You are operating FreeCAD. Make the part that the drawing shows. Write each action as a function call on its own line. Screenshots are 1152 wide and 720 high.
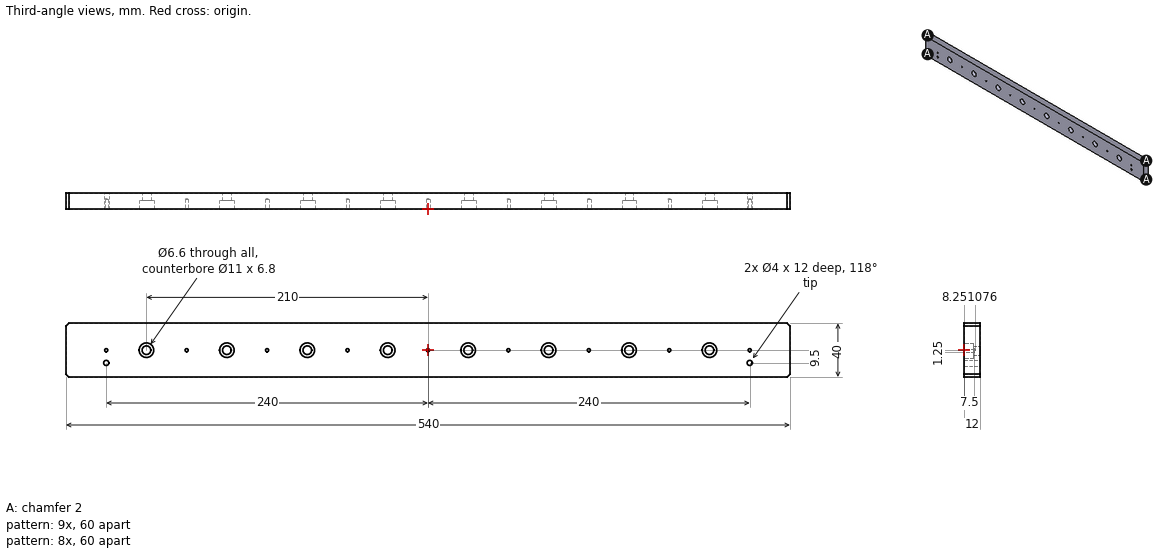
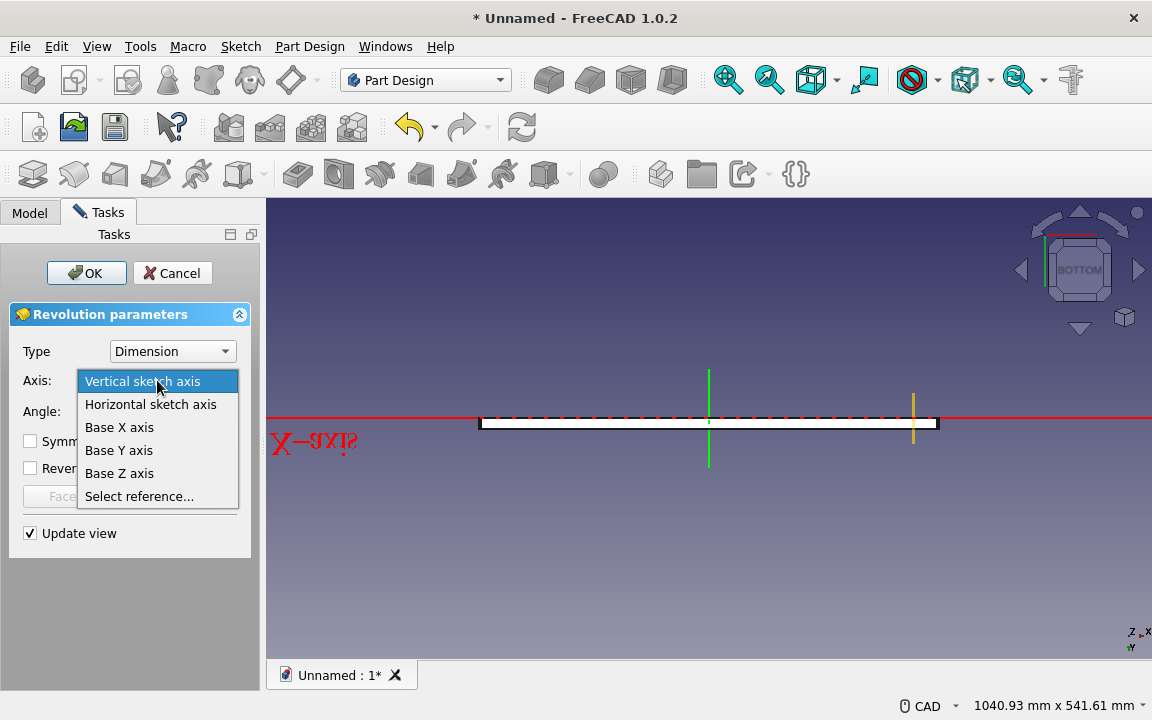
click(156, 404)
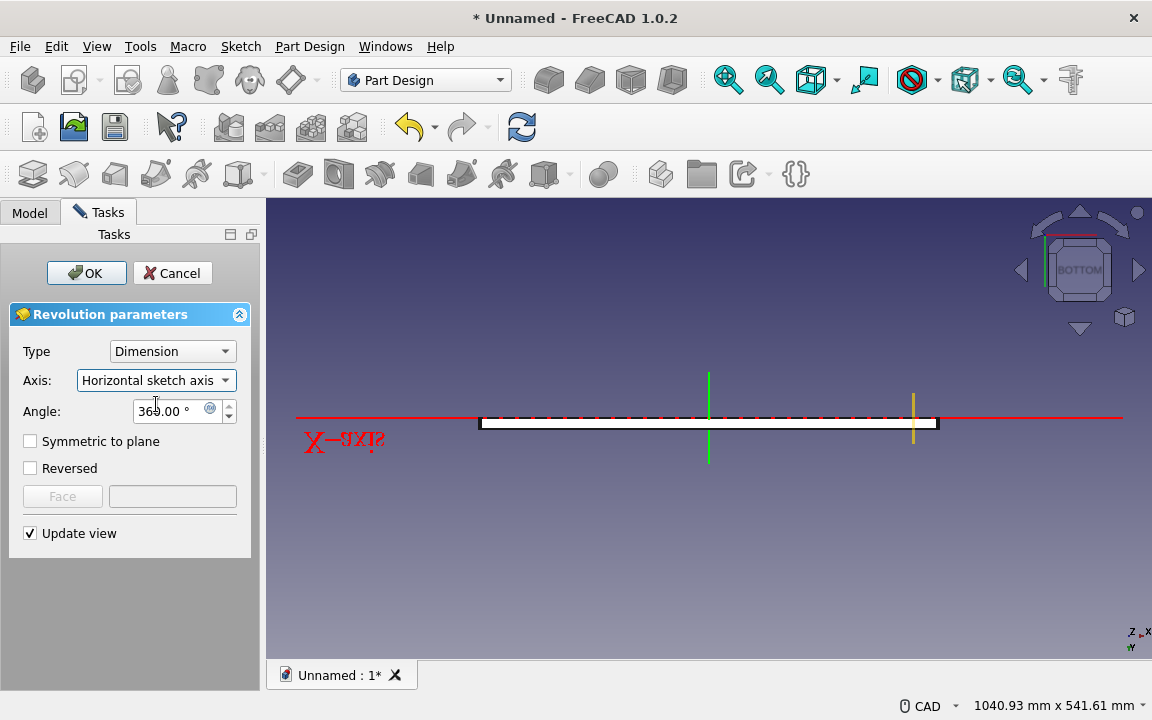
click(87, 273)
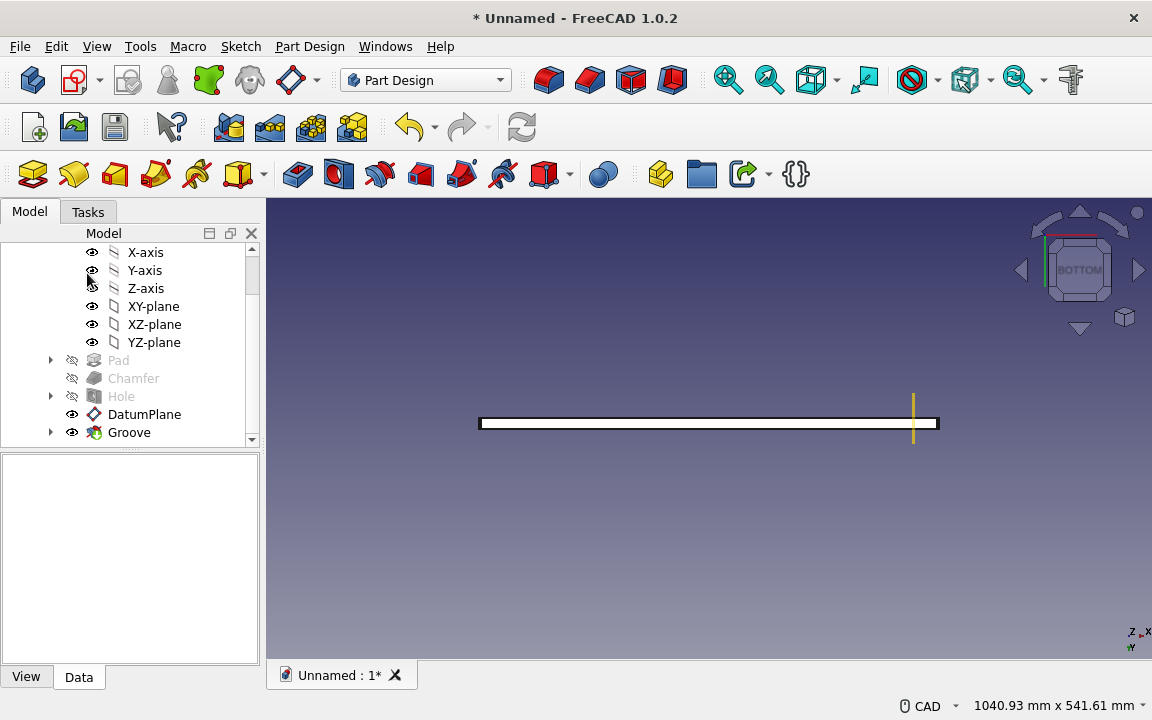
click(117, 414)
key(space)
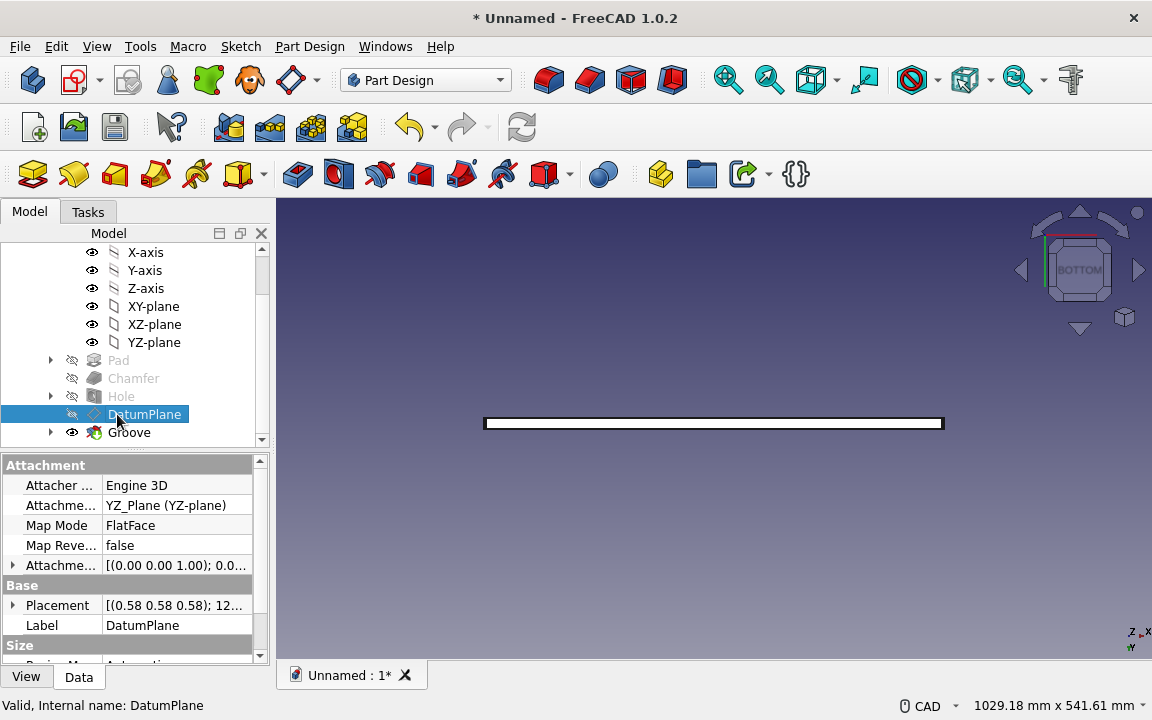
click(117, 432)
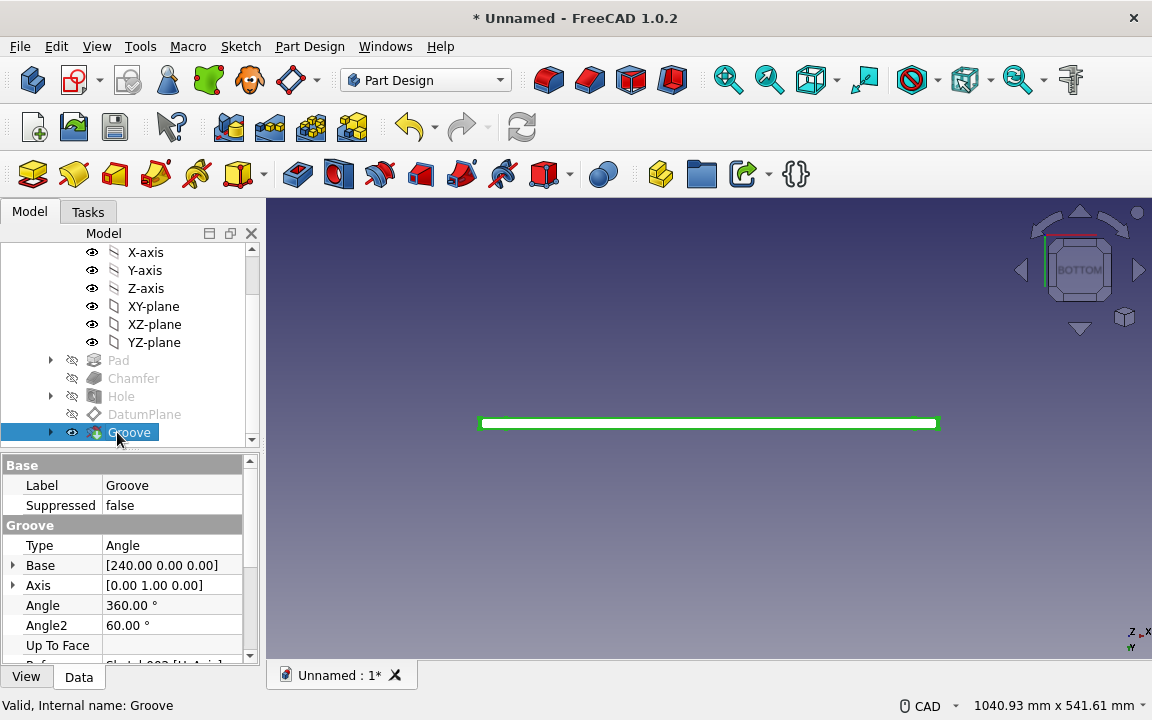
click(270, 128)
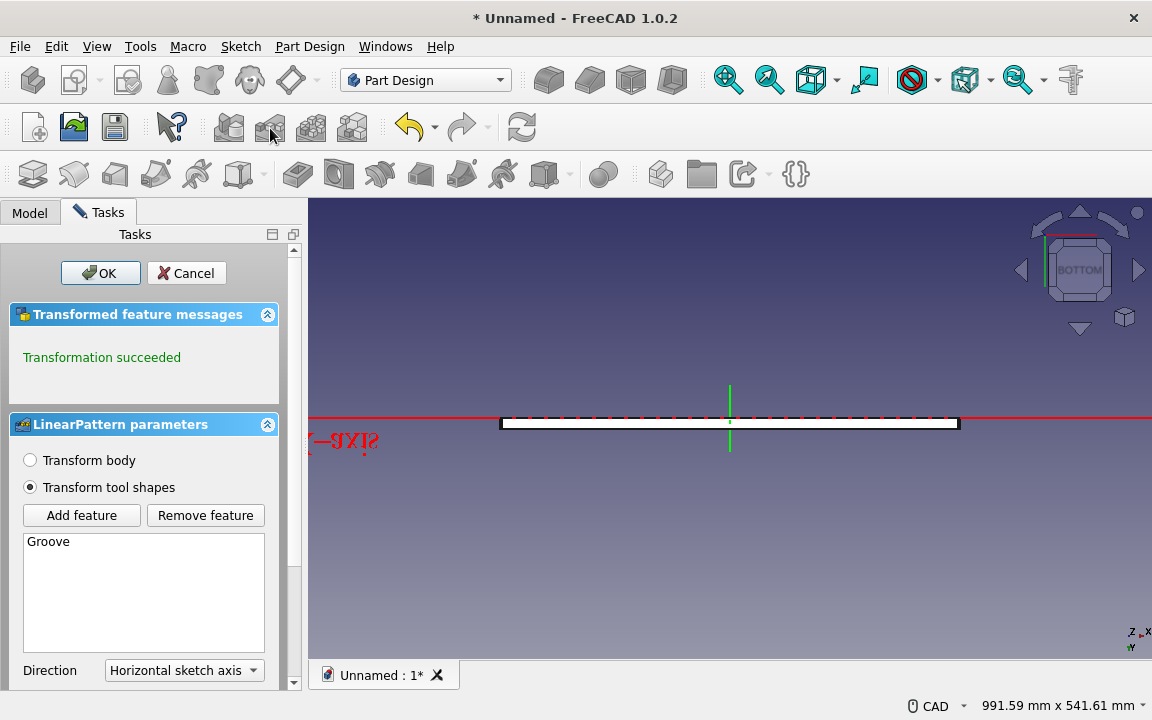
click(185, 670)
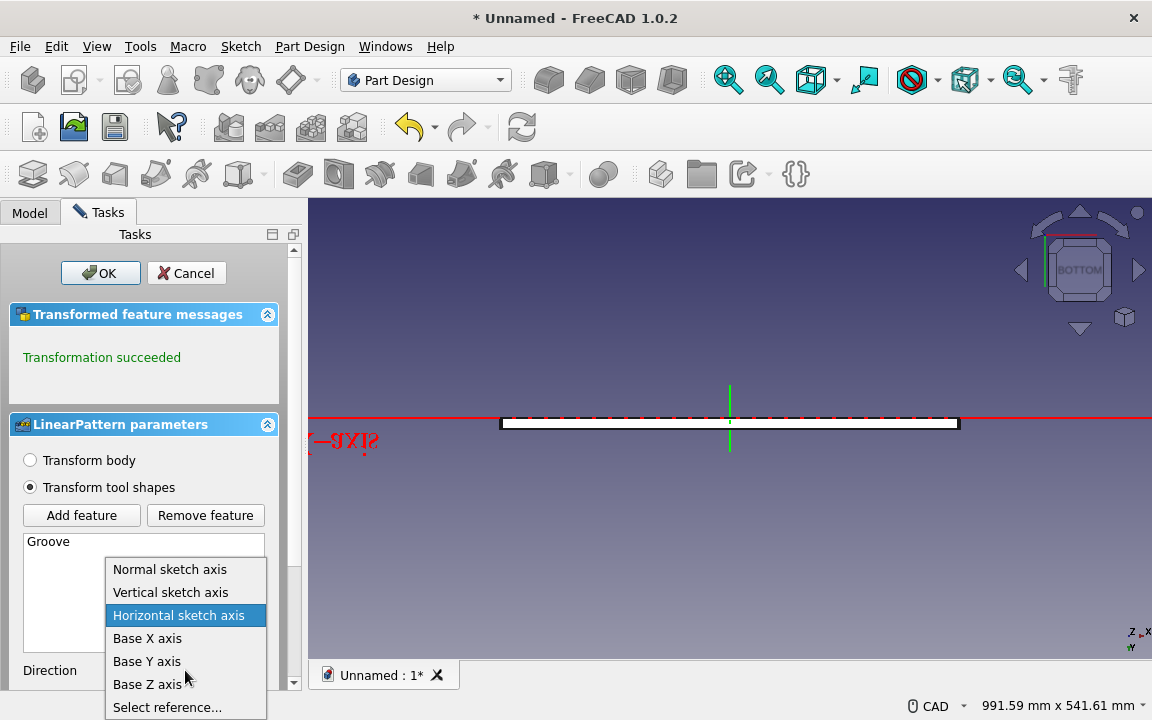
click(184, 638)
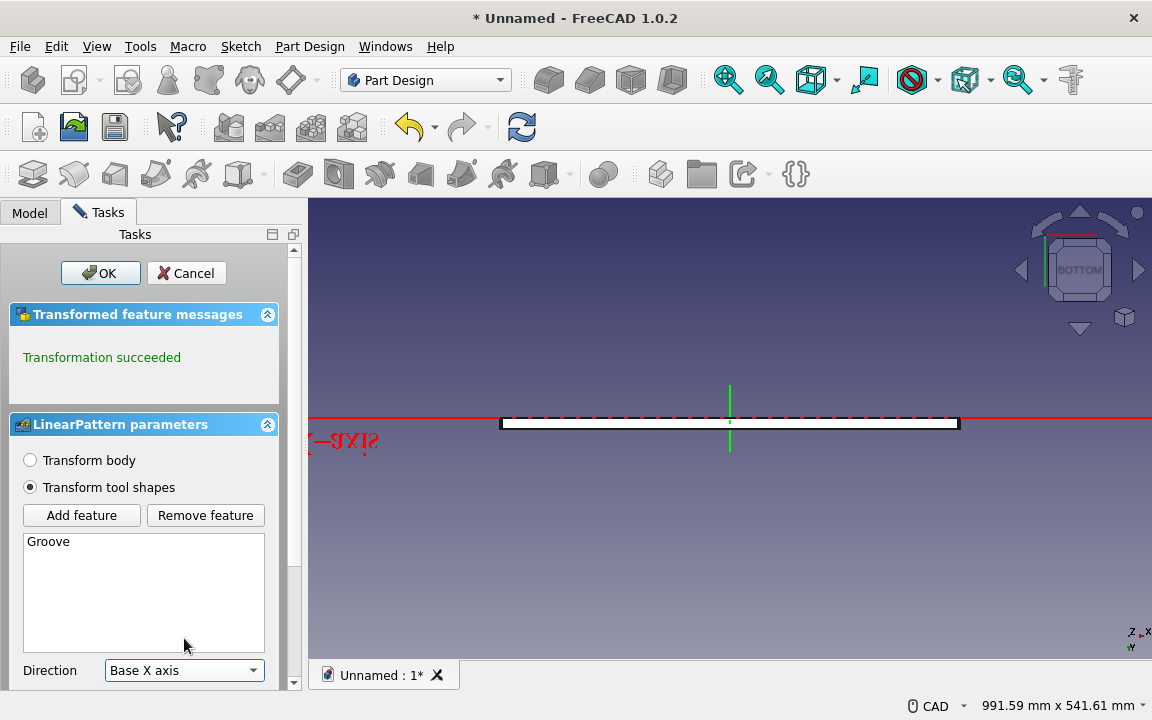
scroll(294, 467, down, 2)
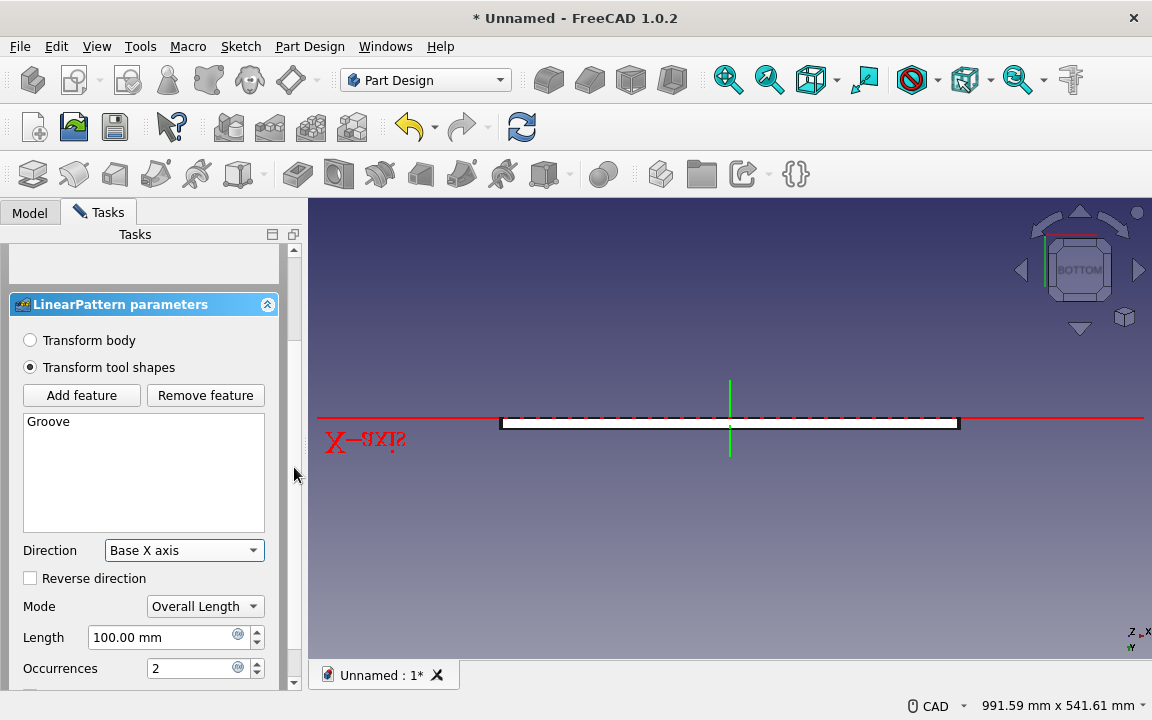
click(206, 606)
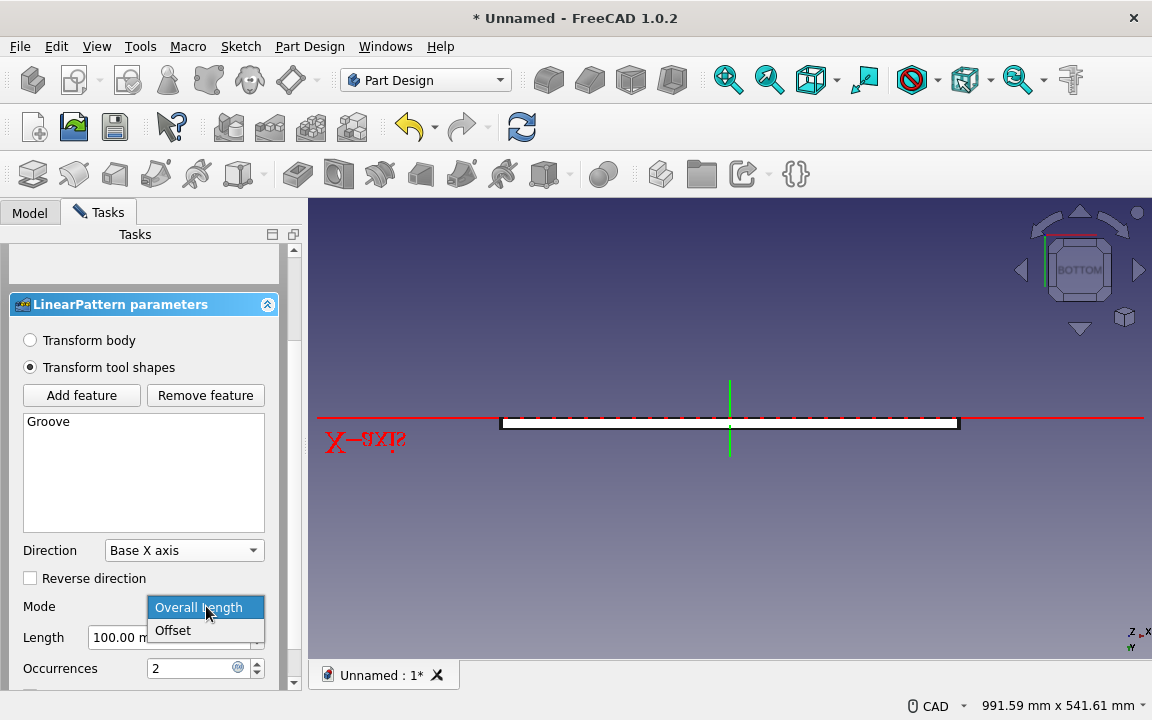
click(204, 630)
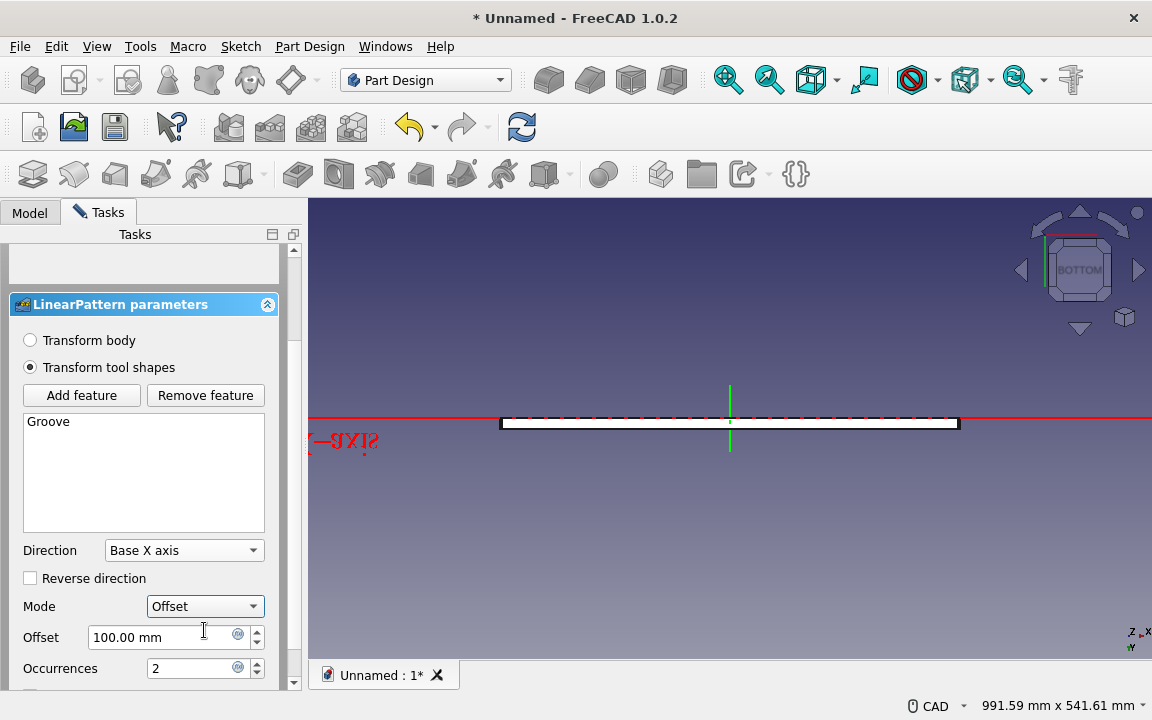
triple_click(170, 638)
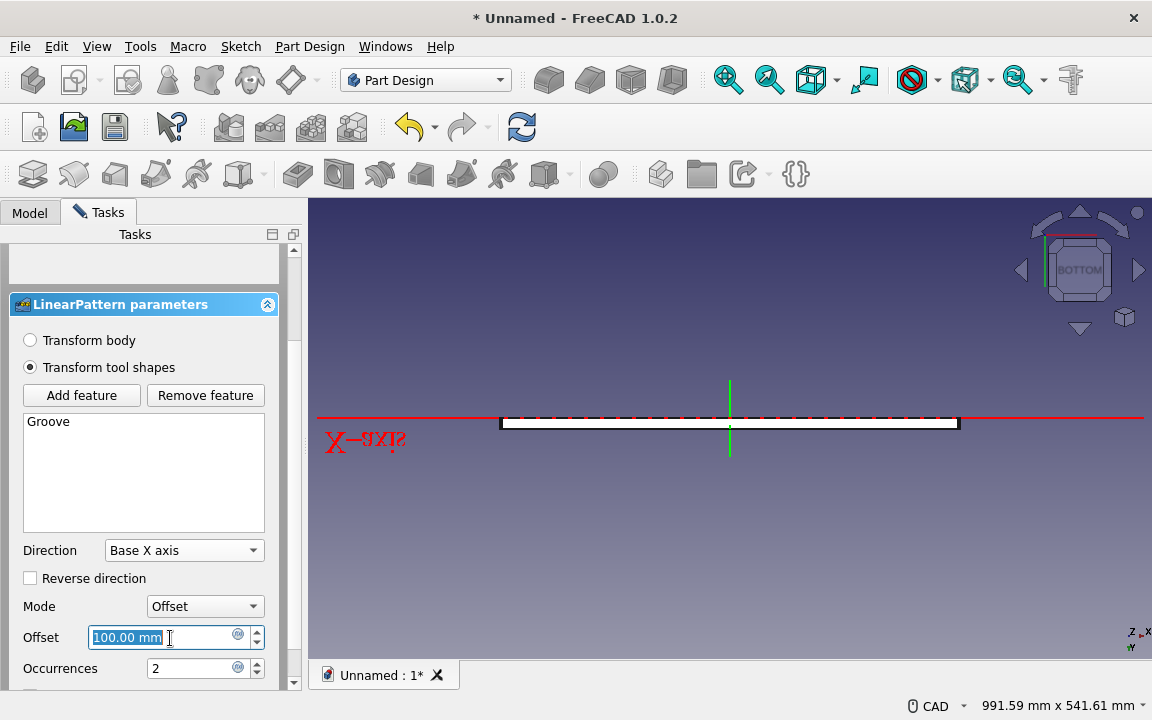
text(60)
key(Tab)